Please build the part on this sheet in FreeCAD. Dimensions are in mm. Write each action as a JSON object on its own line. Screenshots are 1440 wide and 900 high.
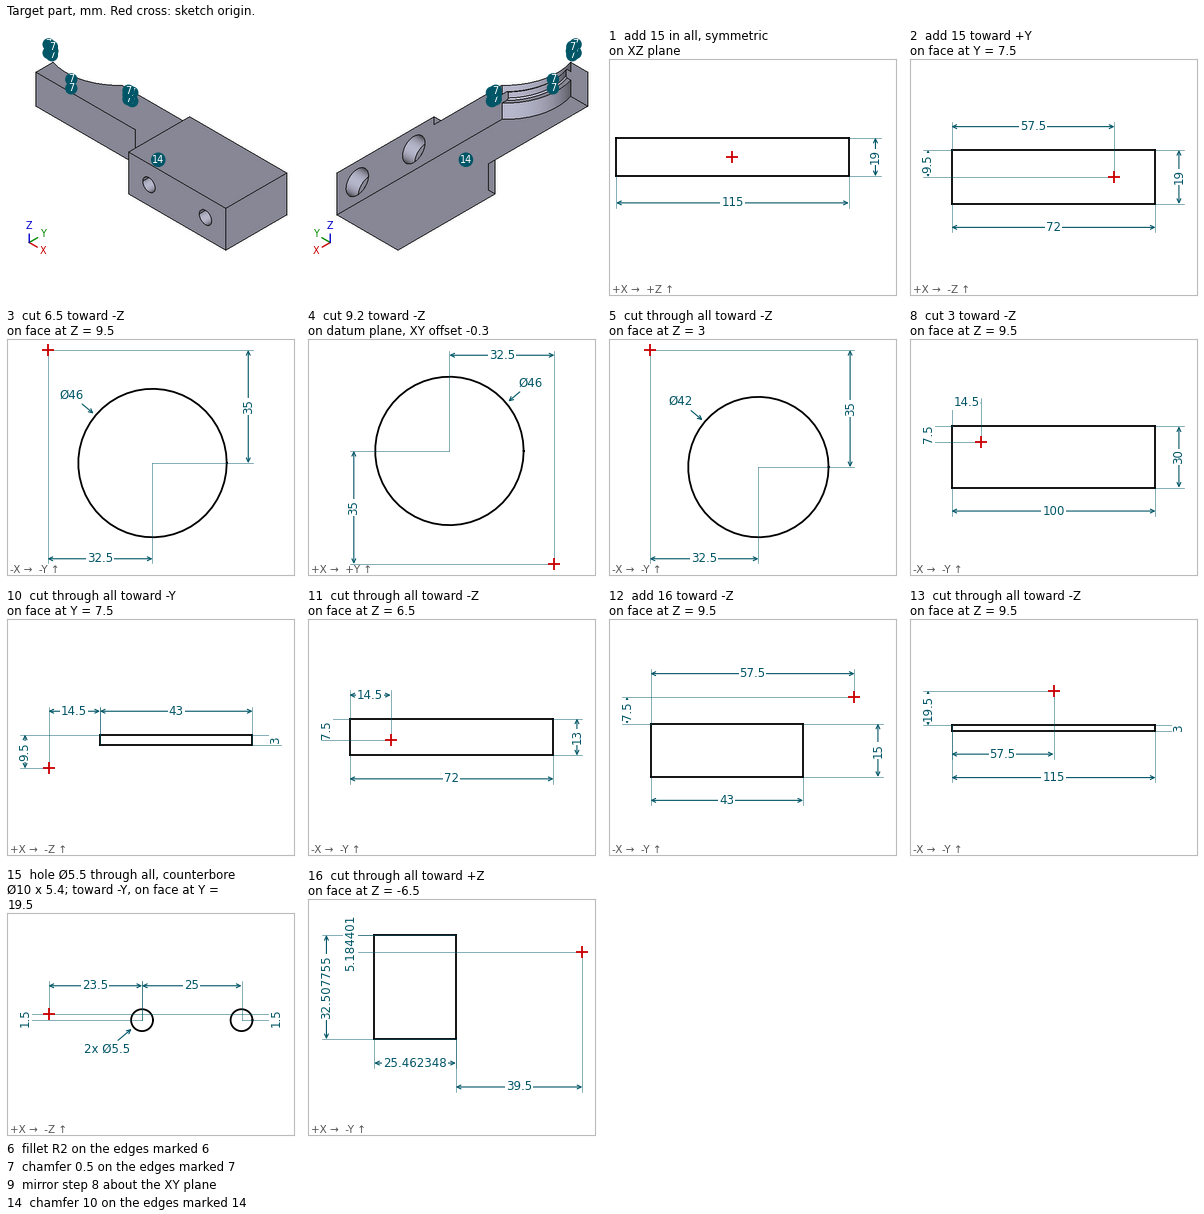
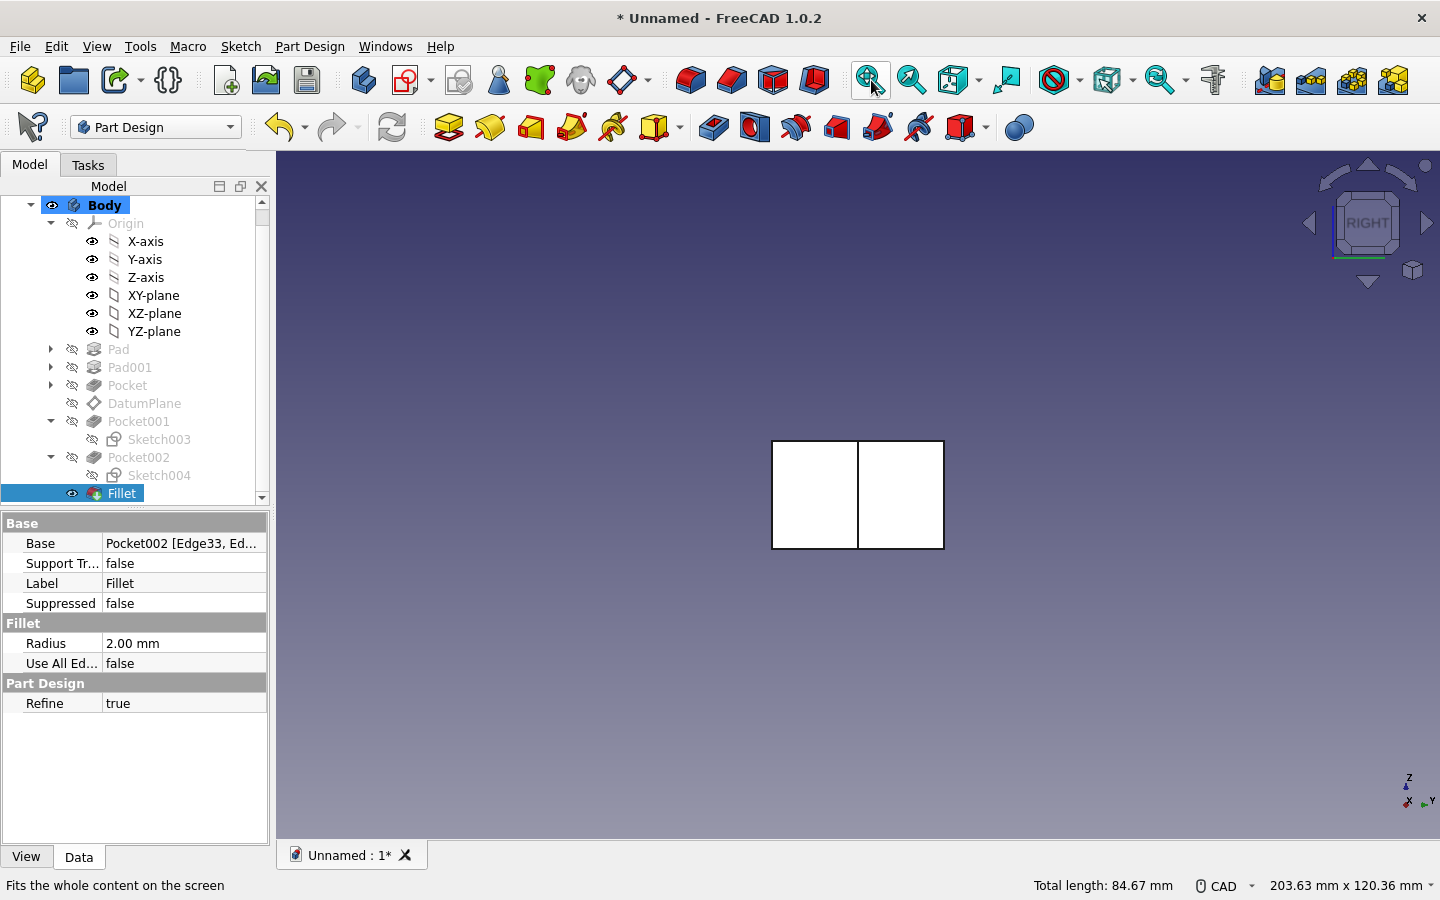
{"action": "scroll", "coordinate": [944, 496], "scroll_direction": "up", "scroll_amount": 8}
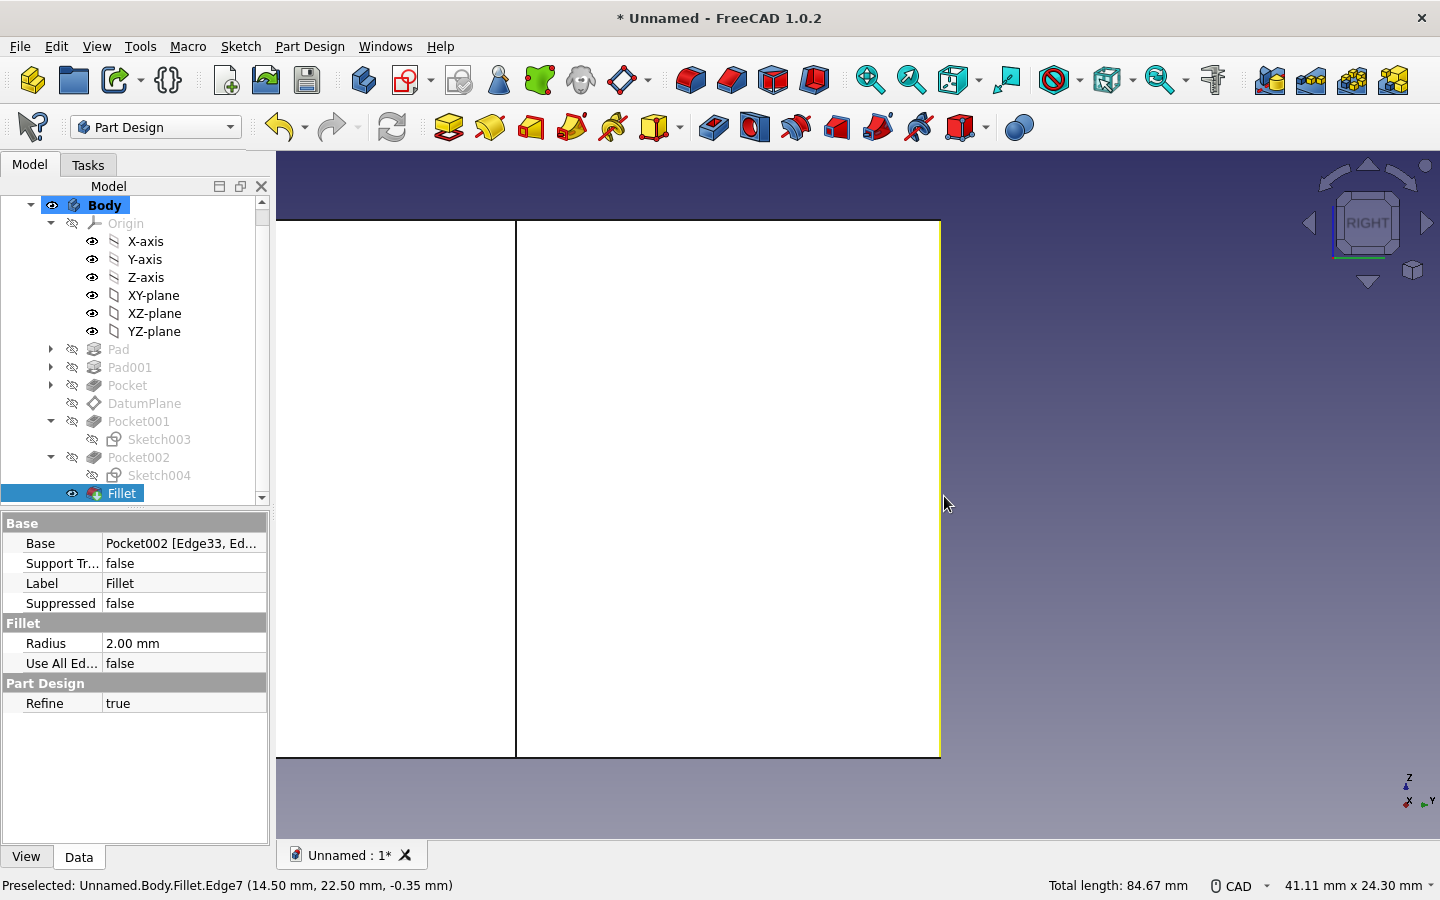
{"action": "left_click", "coordinate": [871, 80]}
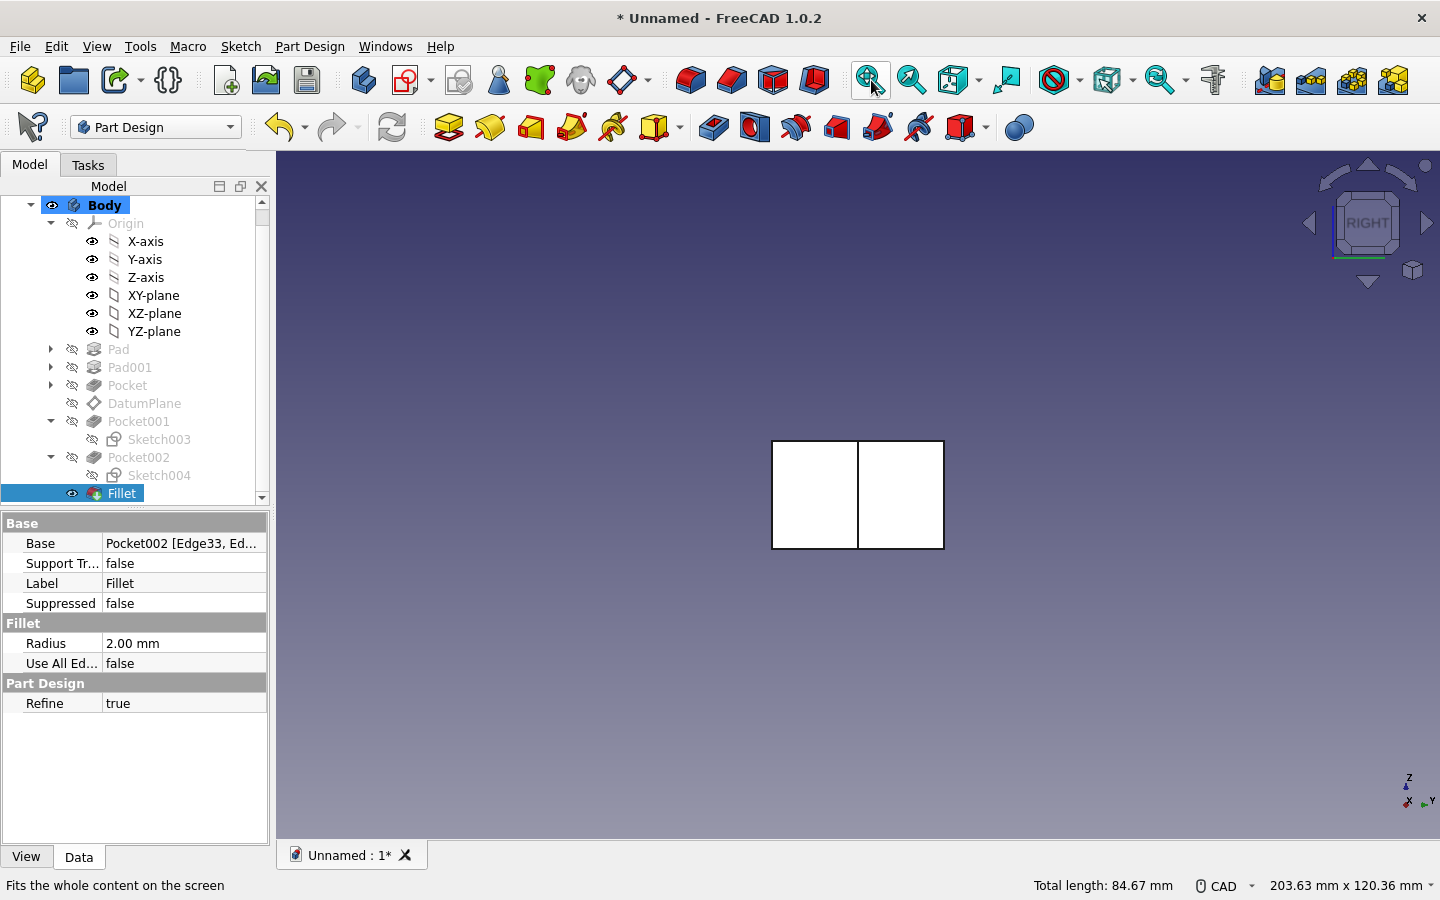
{"action": "key", "text": "5"}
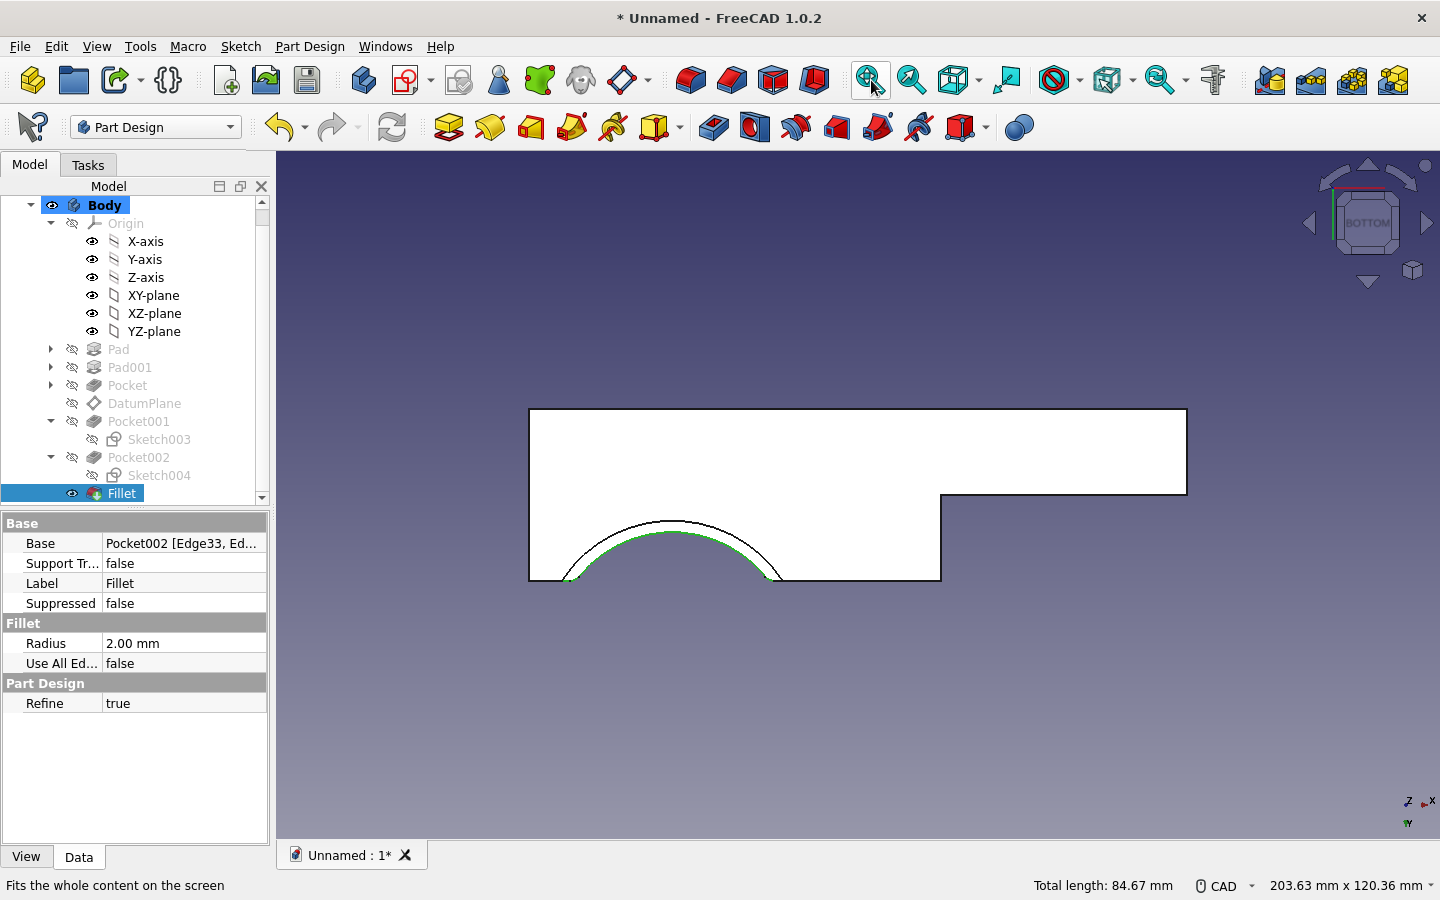
{"action": "scroll", "coordinate": [778, 580], "scroll_direction": "up", "scroll_amount": 8}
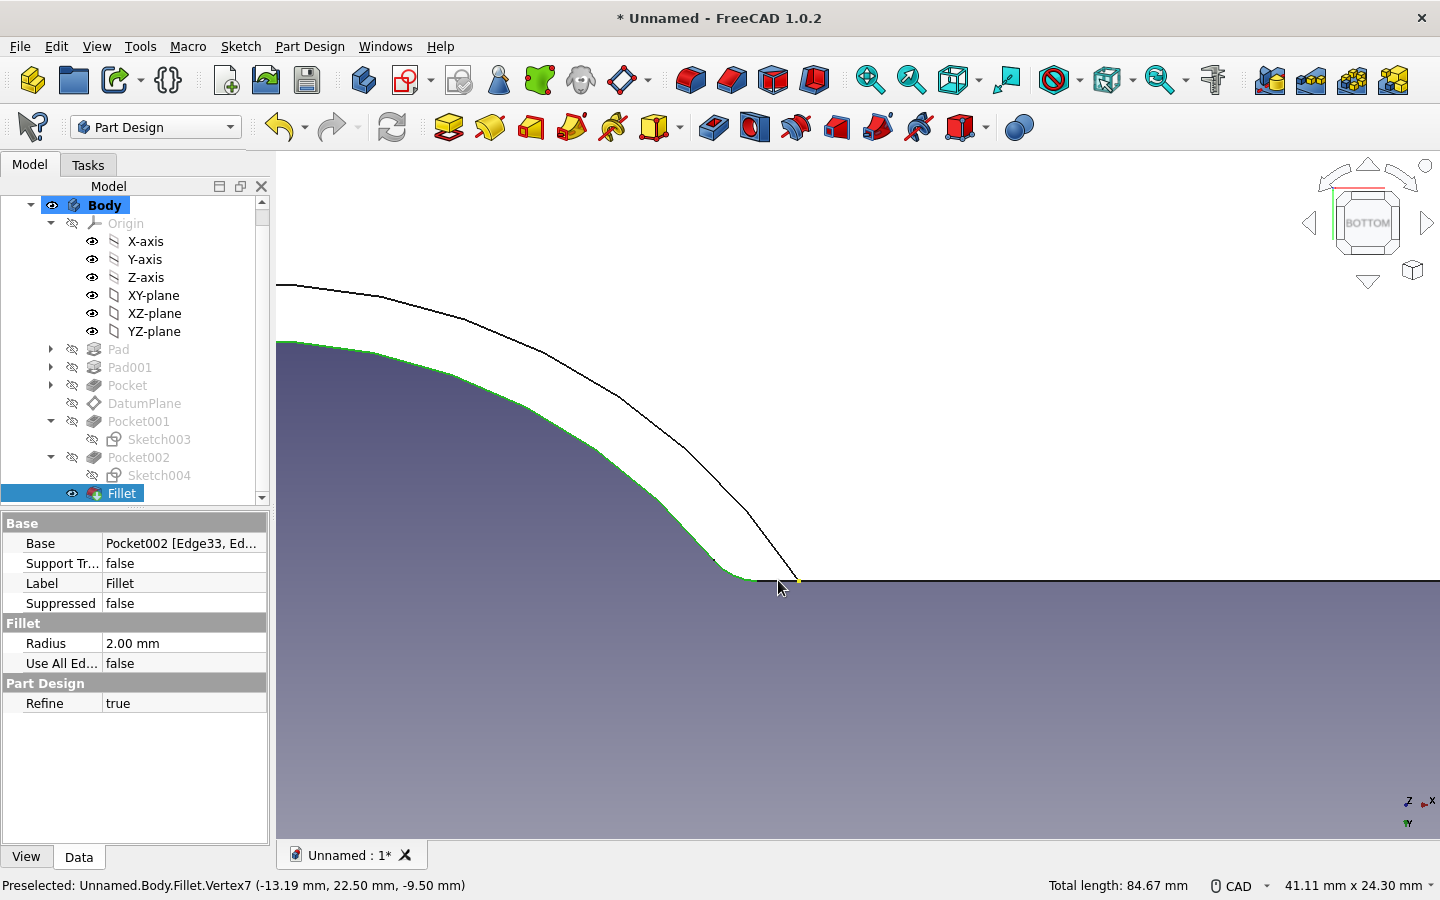
{"action": "left_click", "coordinate": [871, 80]}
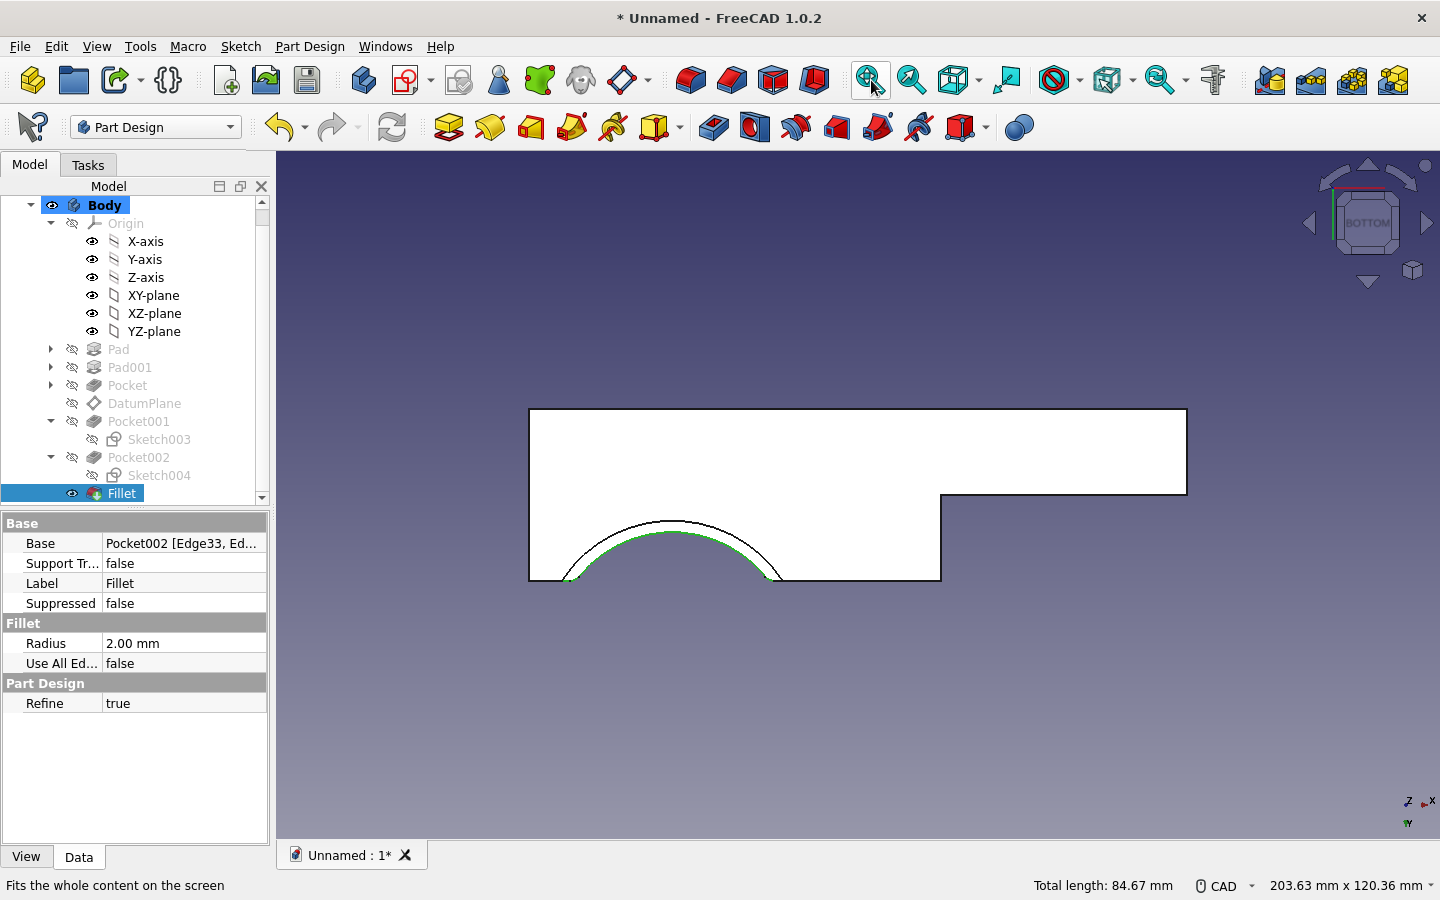
{"action": "key", "text": "4"}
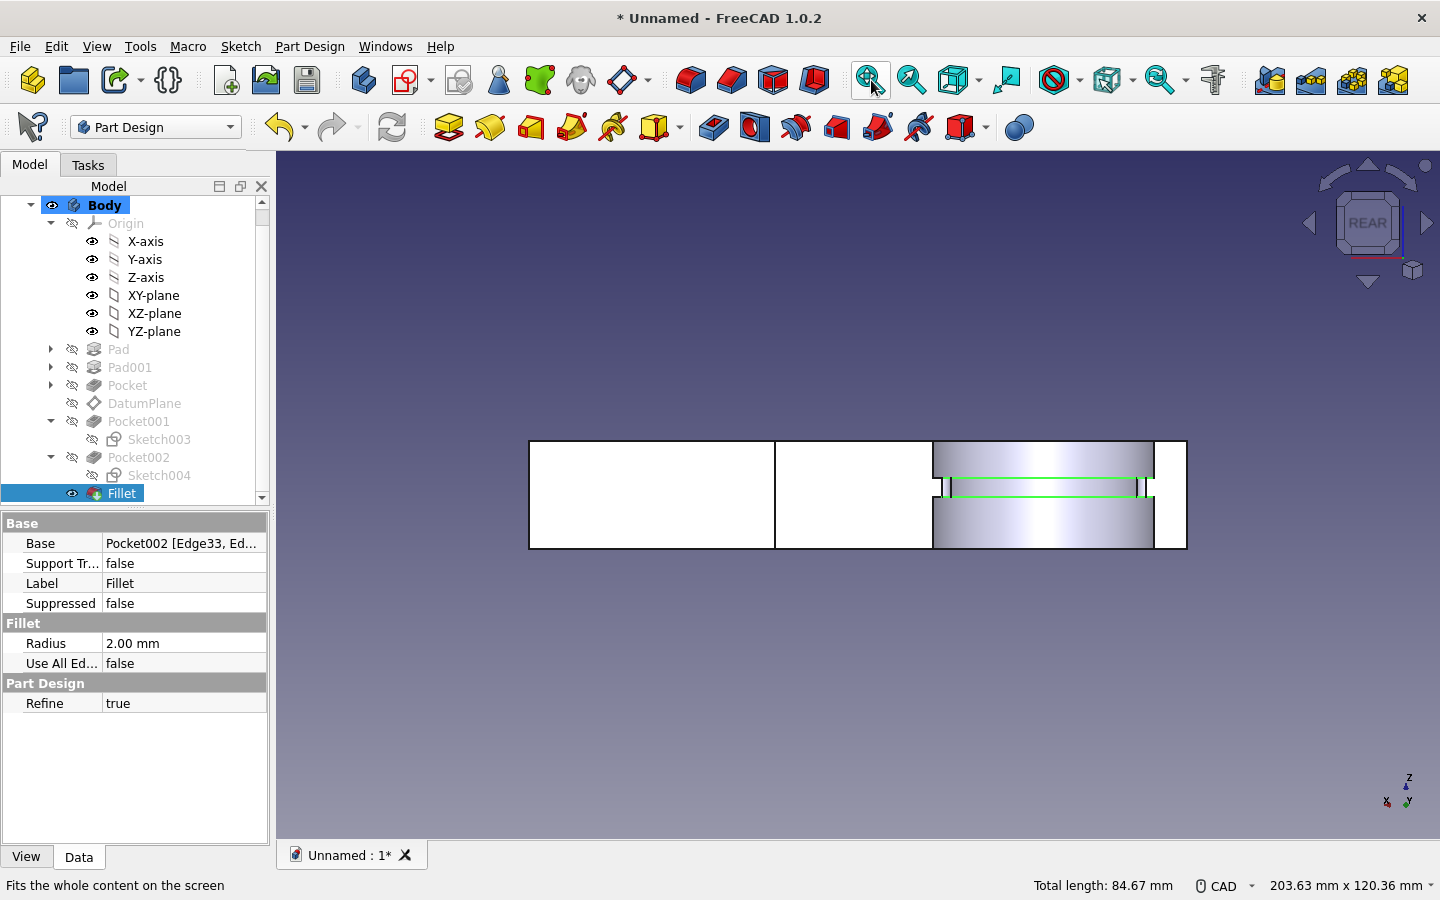
{"action": "scroll", "coordinate": [938, 496], "scroll_direction": "up", "scroll_amount": 8}